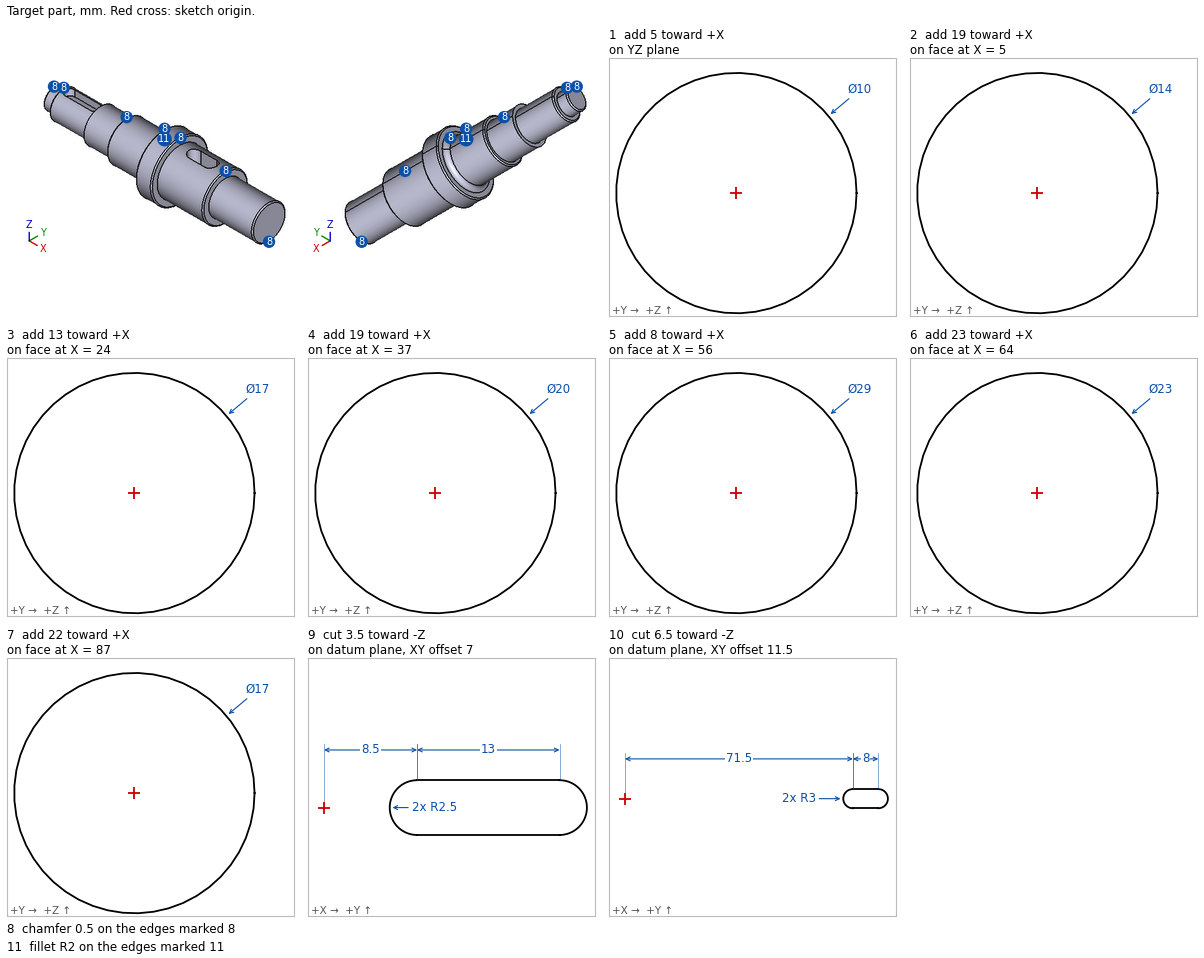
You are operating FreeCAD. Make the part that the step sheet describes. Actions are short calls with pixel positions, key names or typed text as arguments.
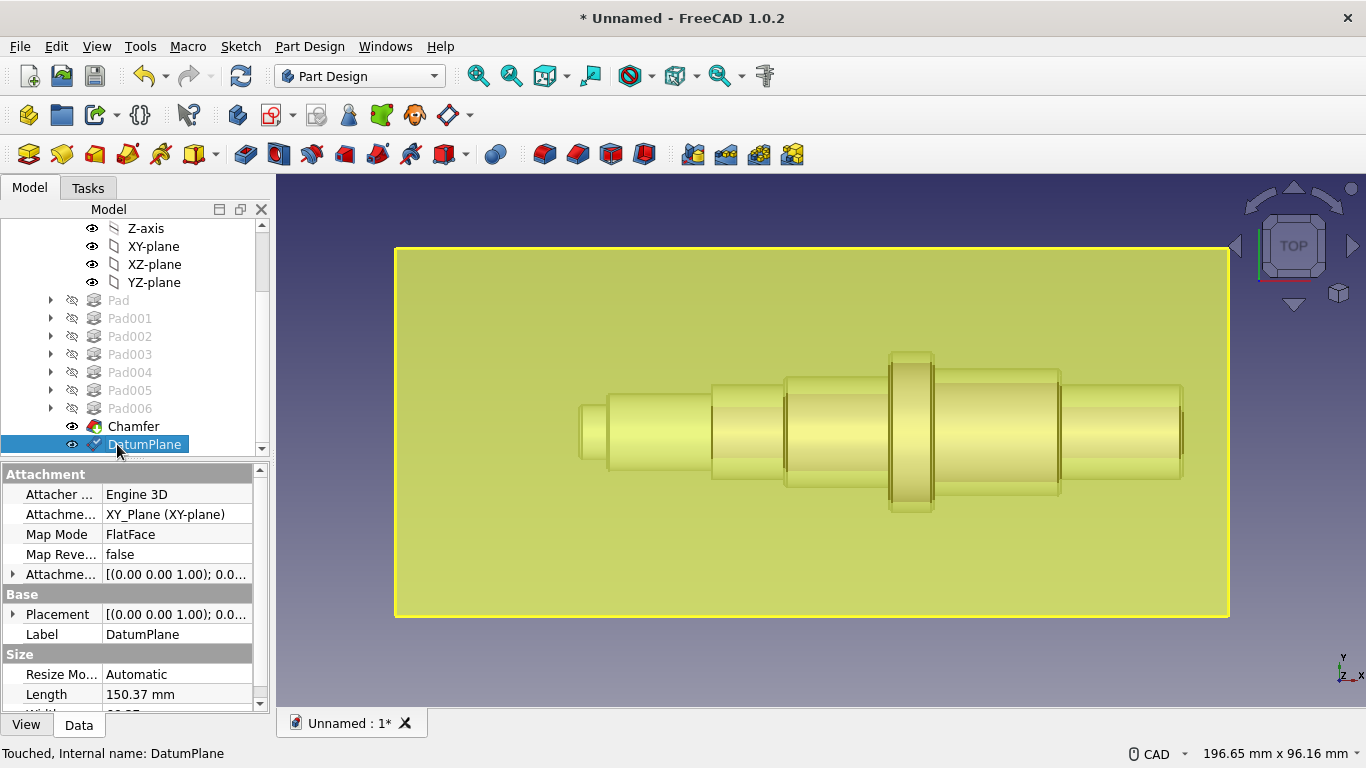
click(270, 116)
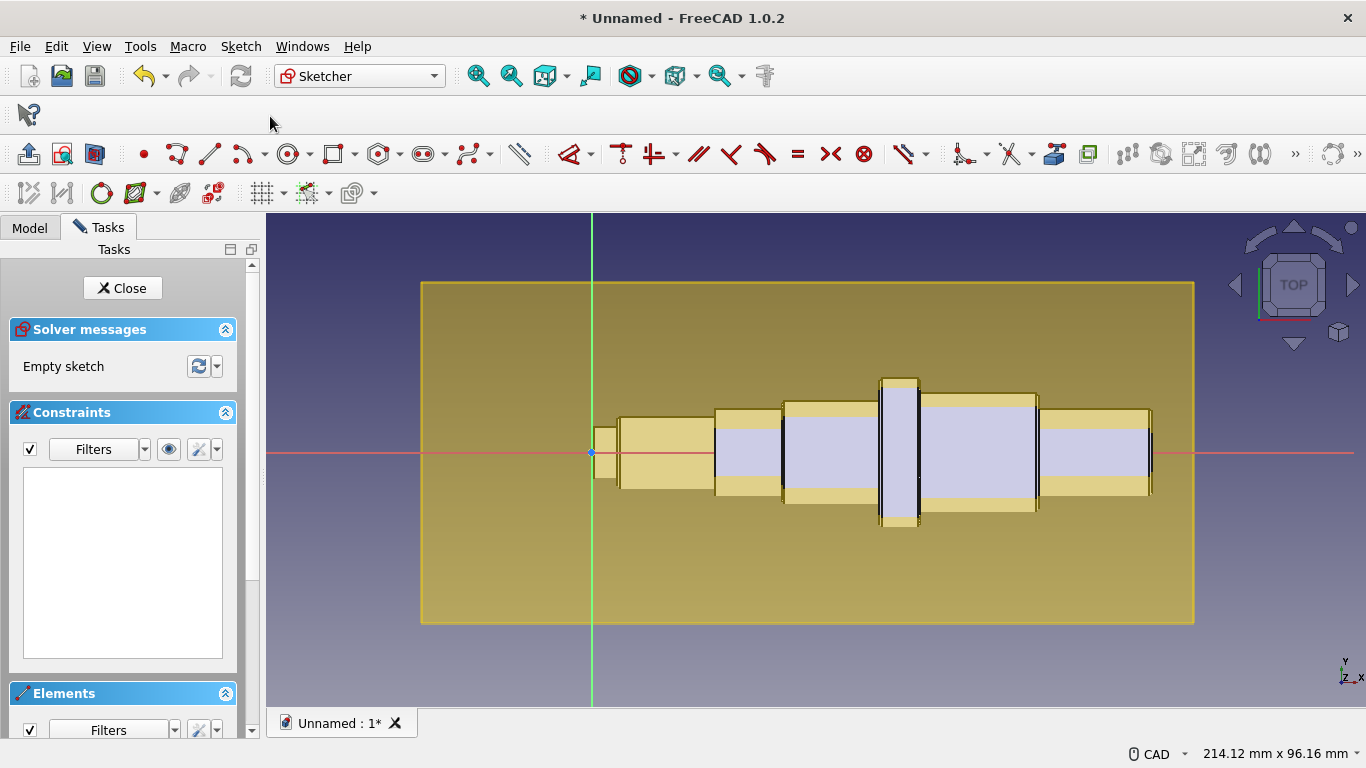
click(95, 154)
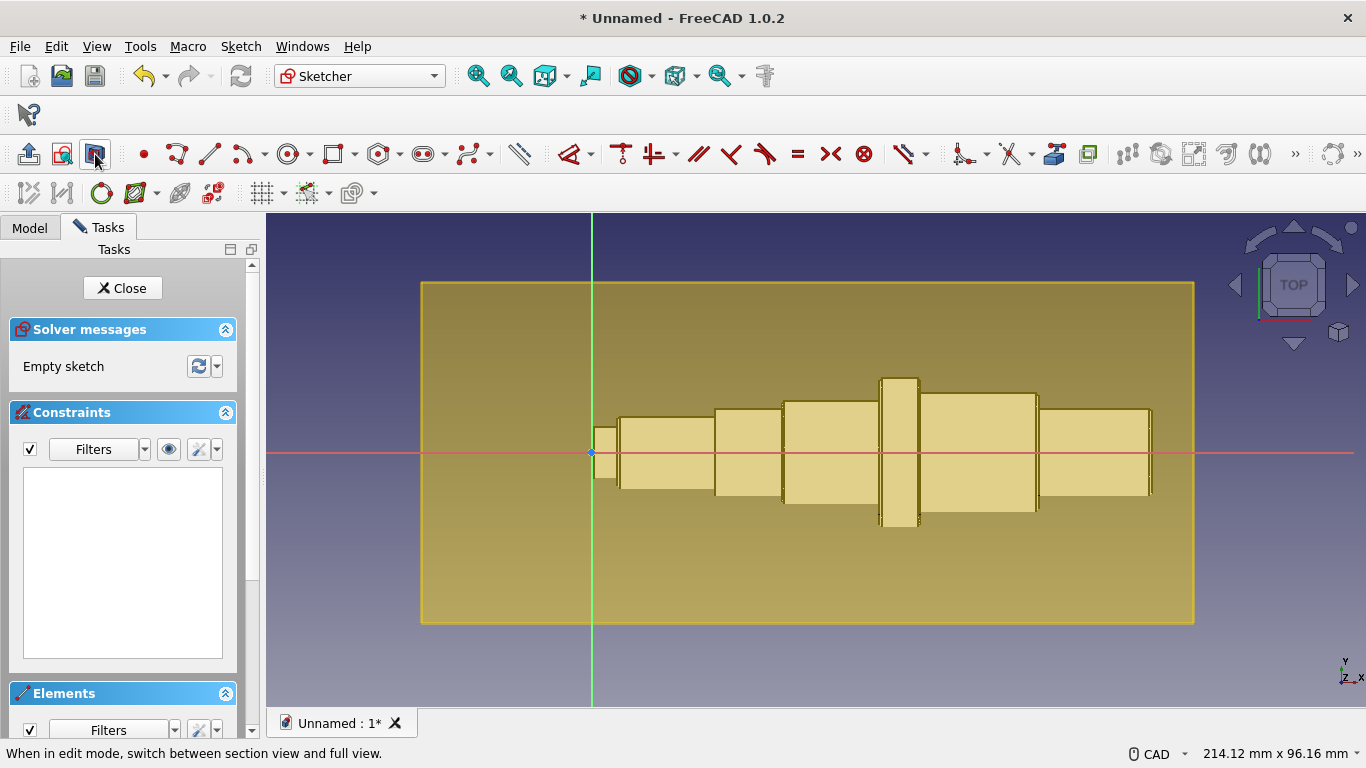
scroll(630, 451, up, 8)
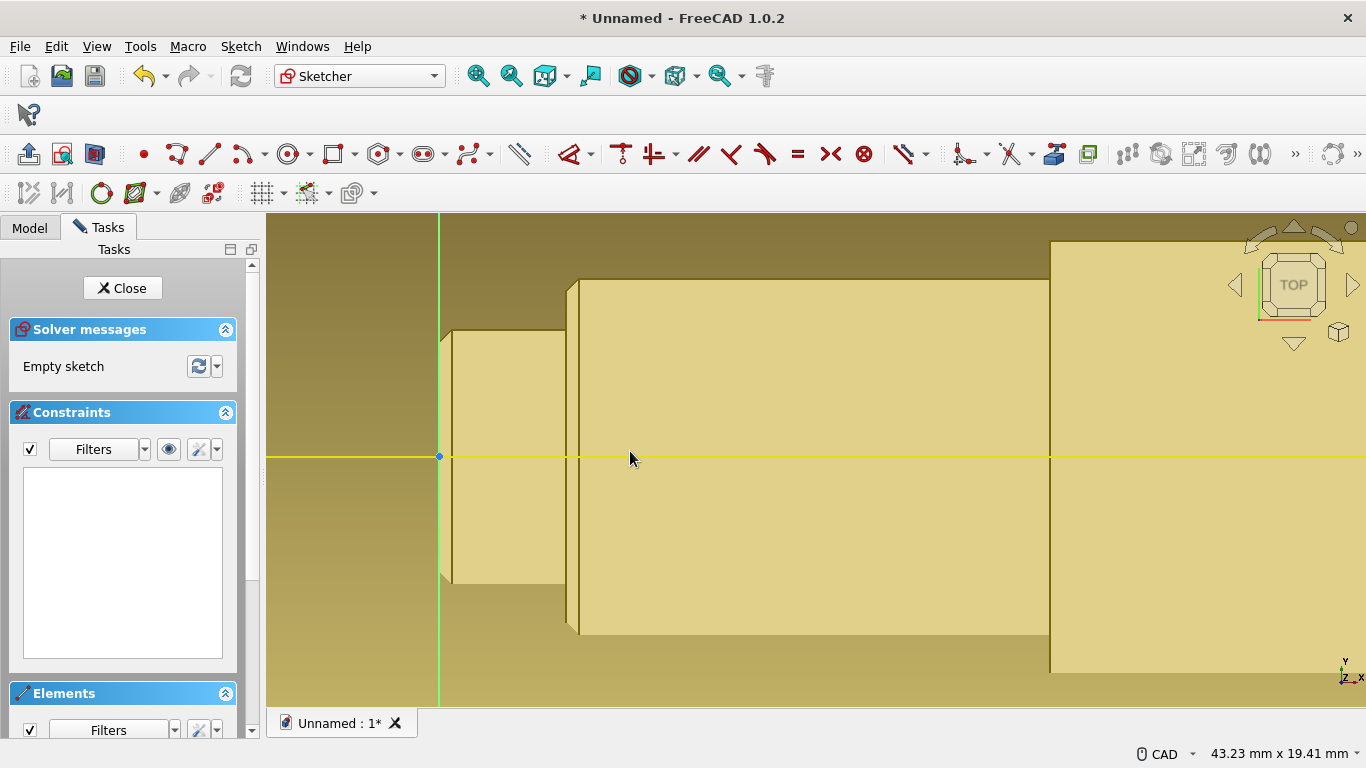
click(422, 154)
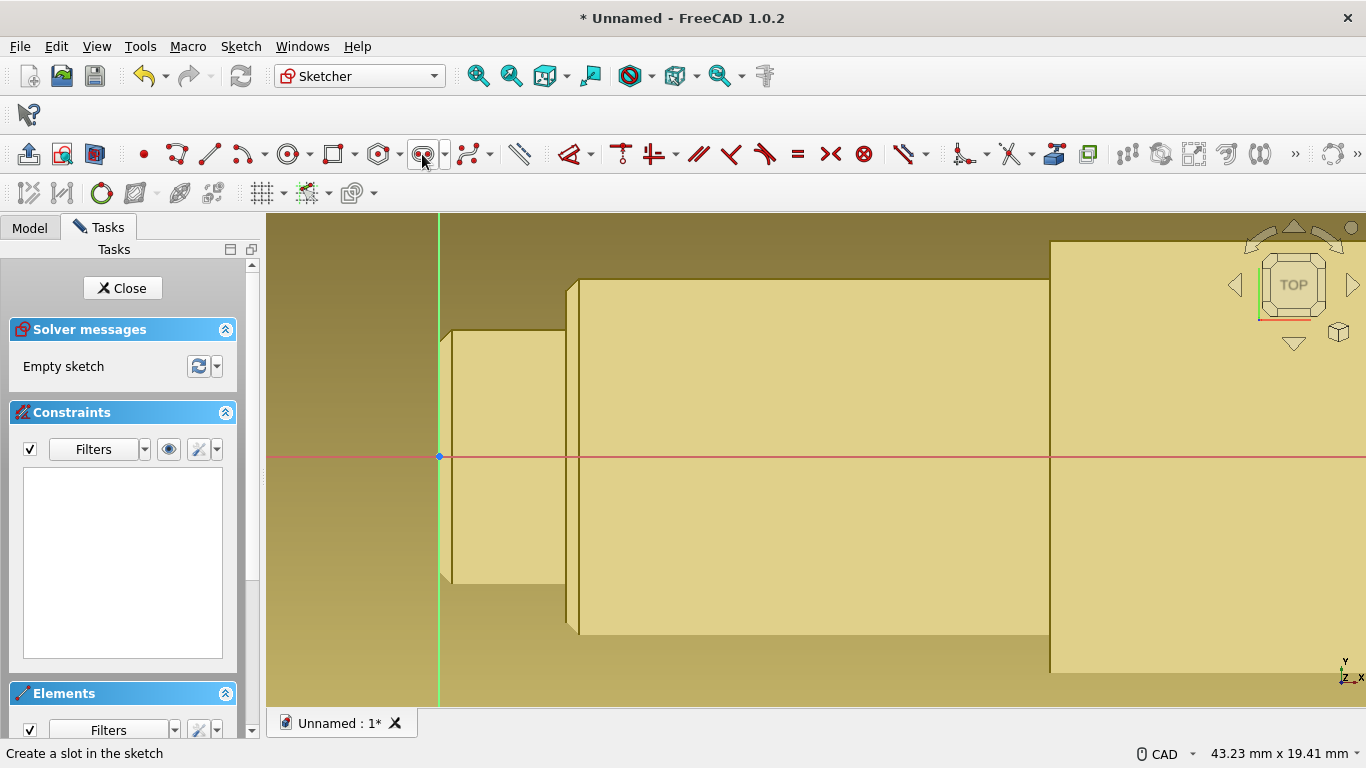
click(655, 457)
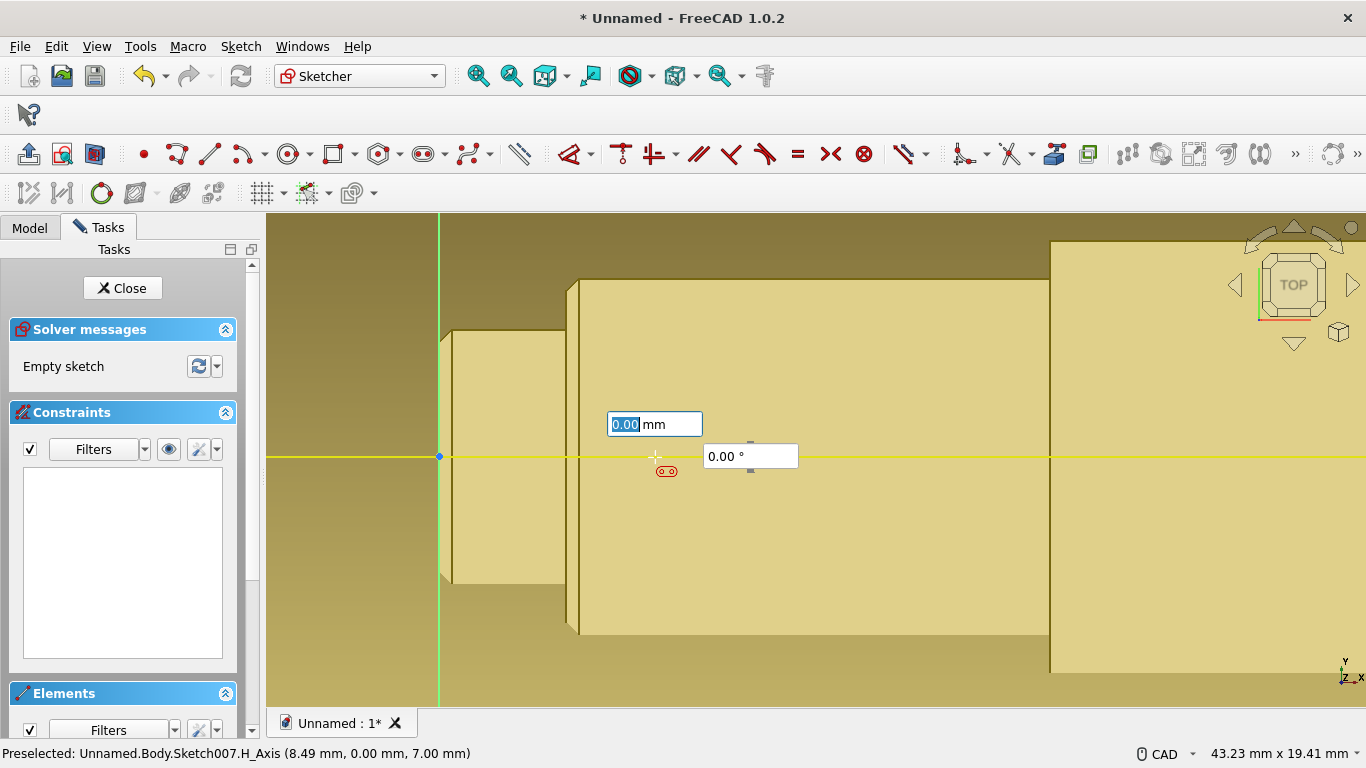
click(986, 448)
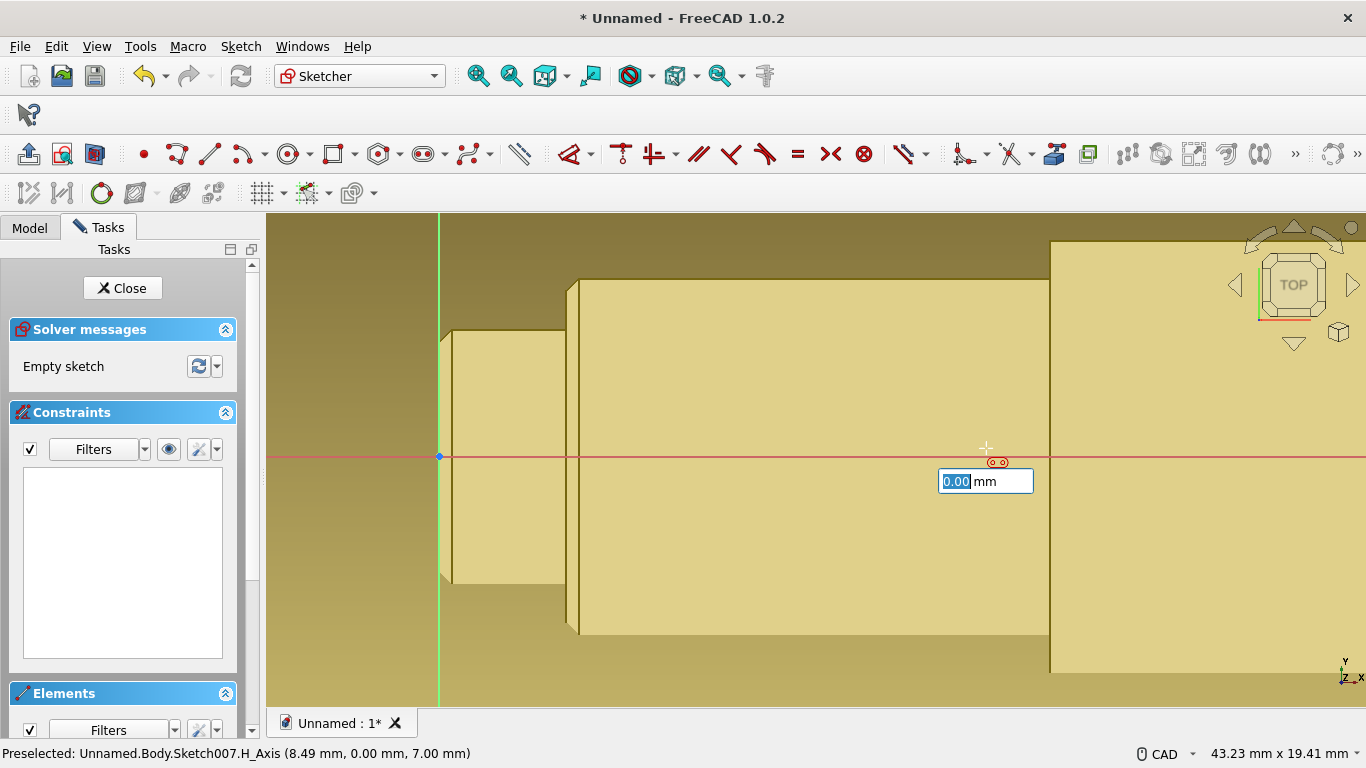
click(821, 393)
key(Escape)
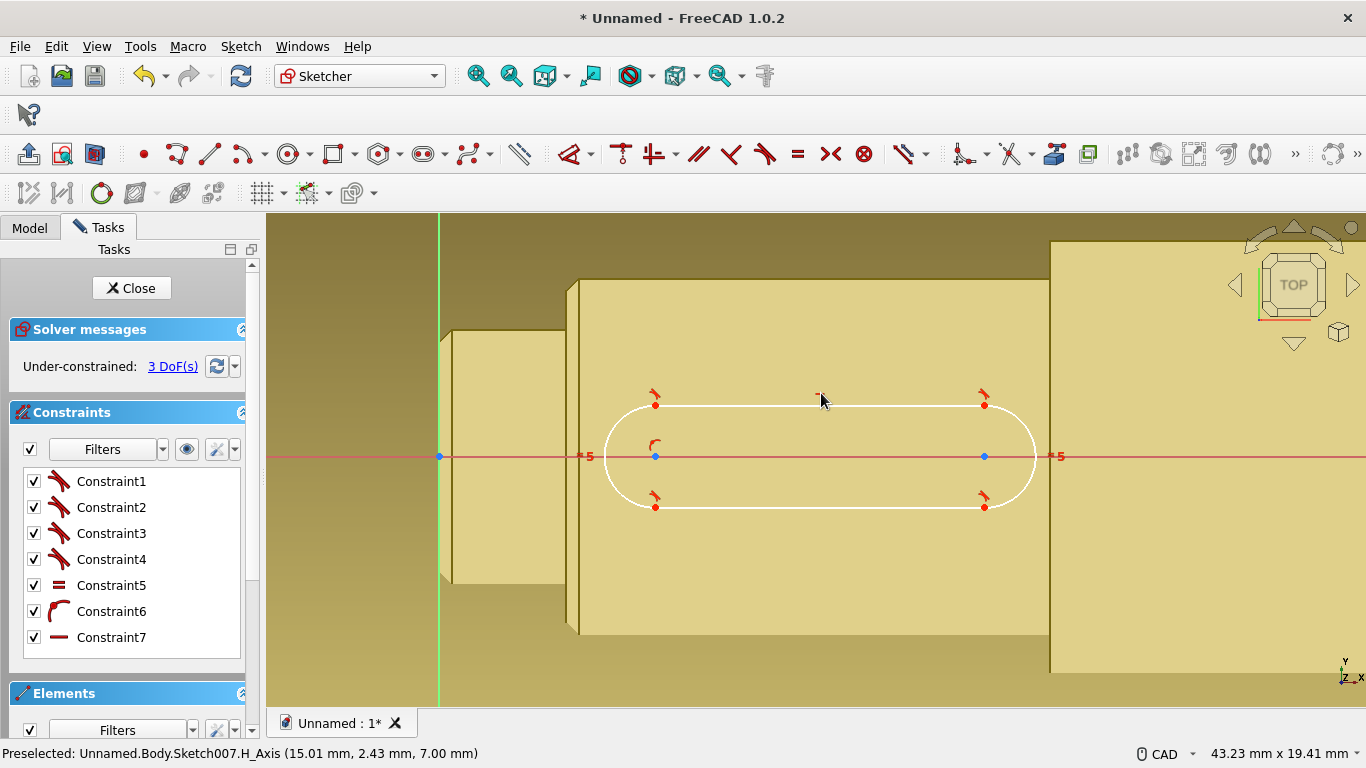
click(568, 154)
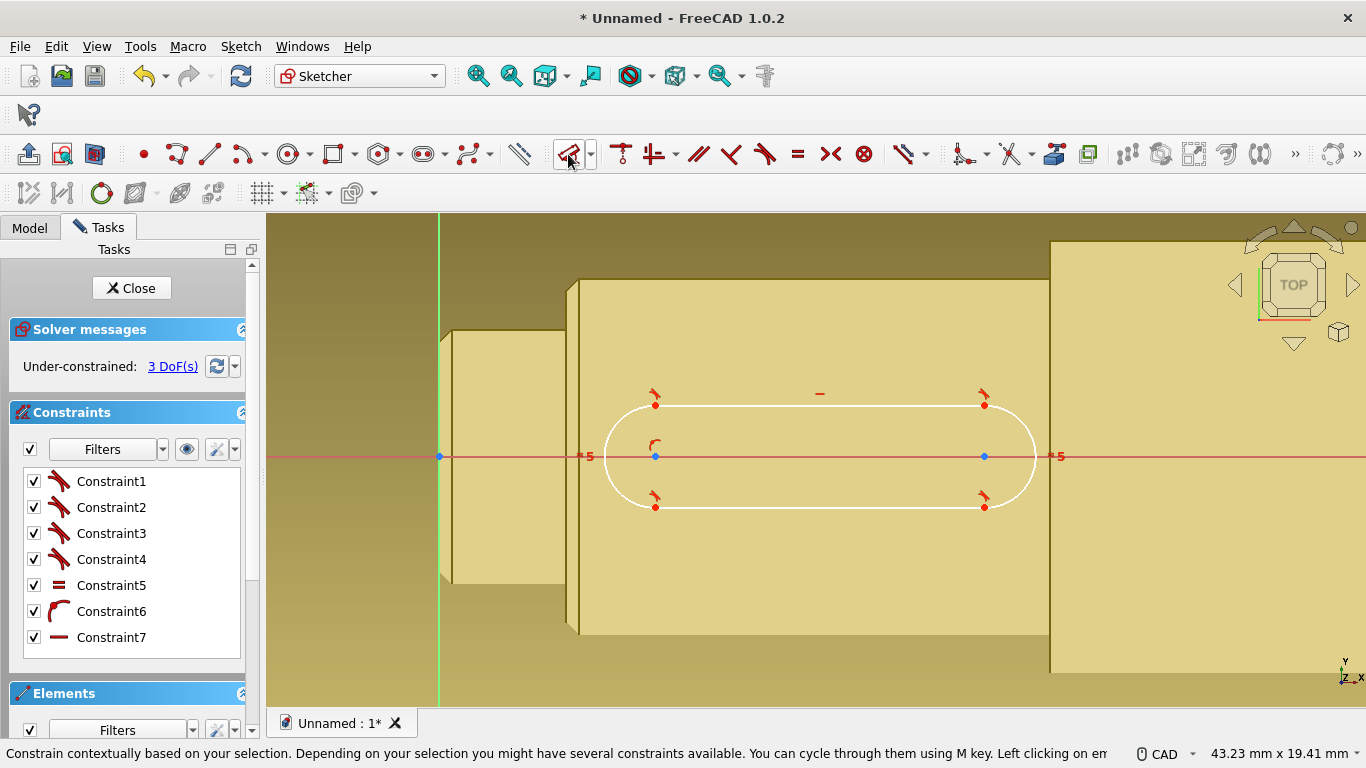
click(614, 427)
click(588, 408)